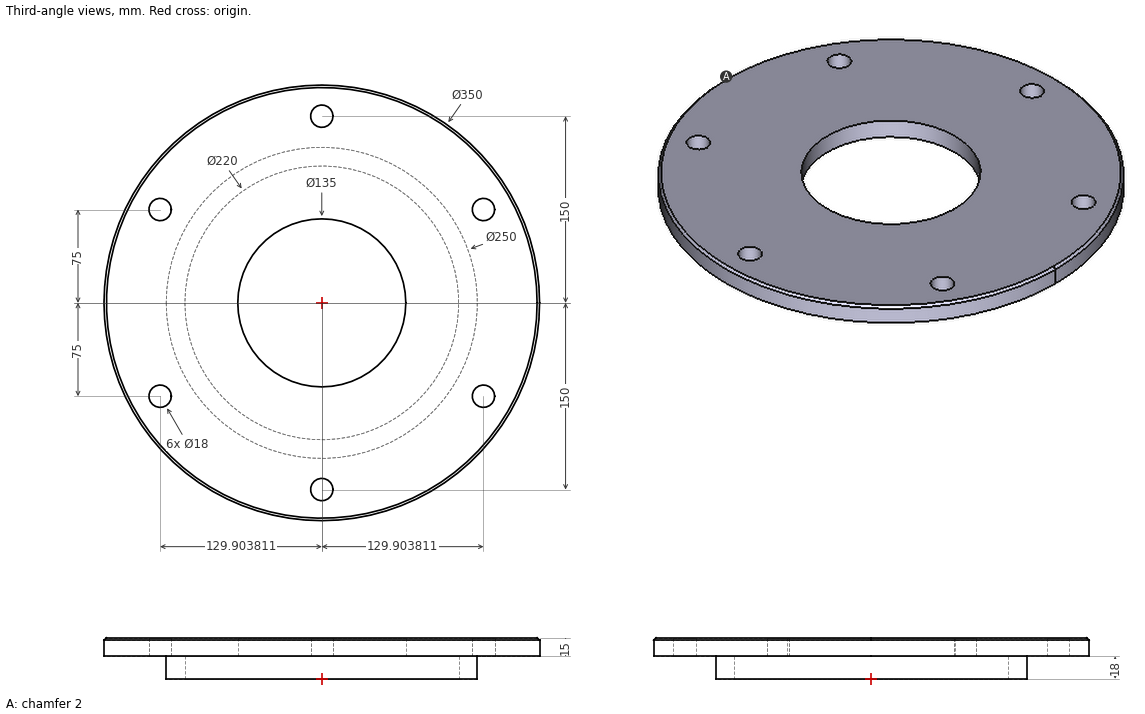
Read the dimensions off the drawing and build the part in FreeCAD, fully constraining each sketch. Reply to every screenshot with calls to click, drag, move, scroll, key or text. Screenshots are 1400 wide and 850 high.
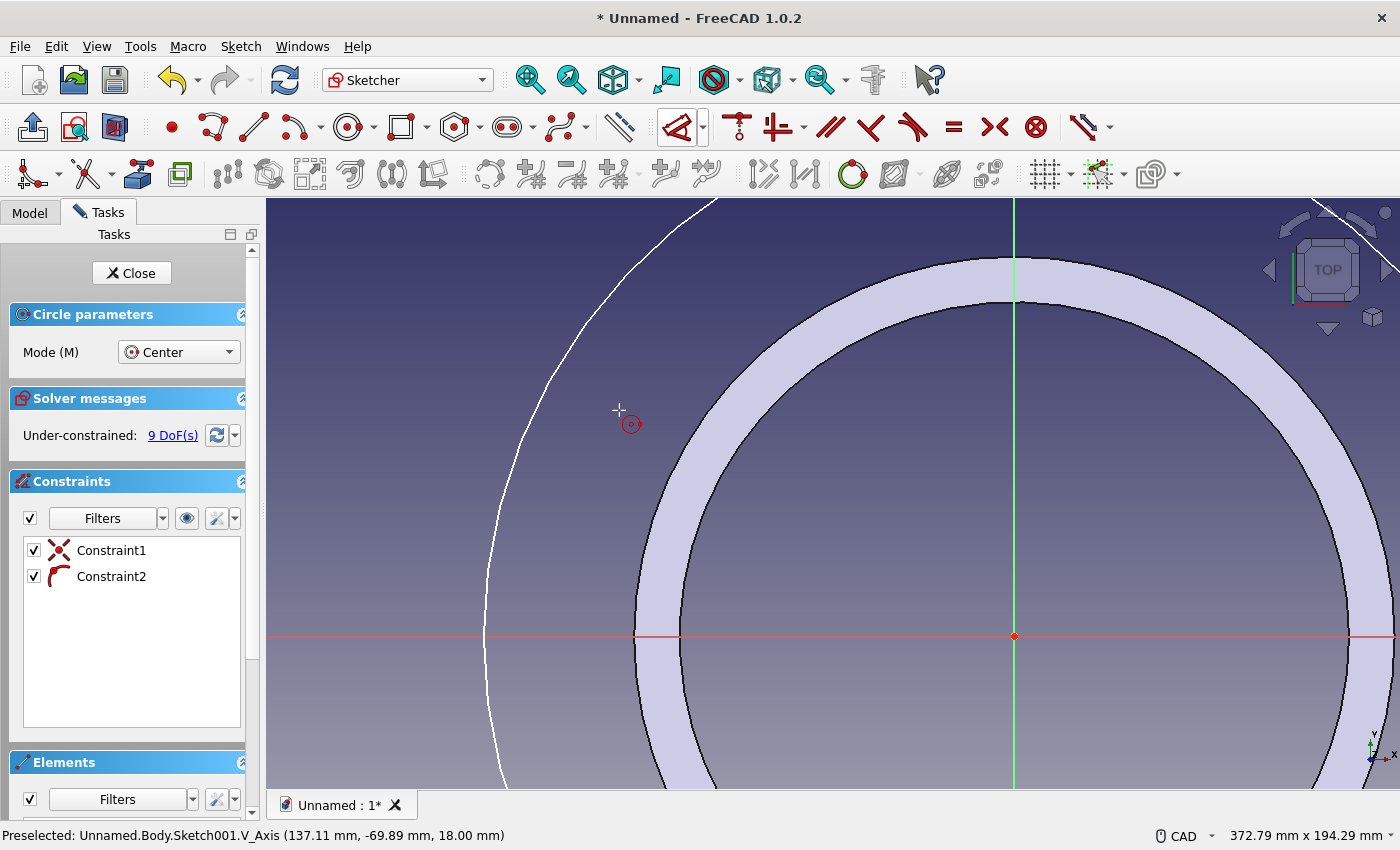
click(619, 409)
click(639, 389)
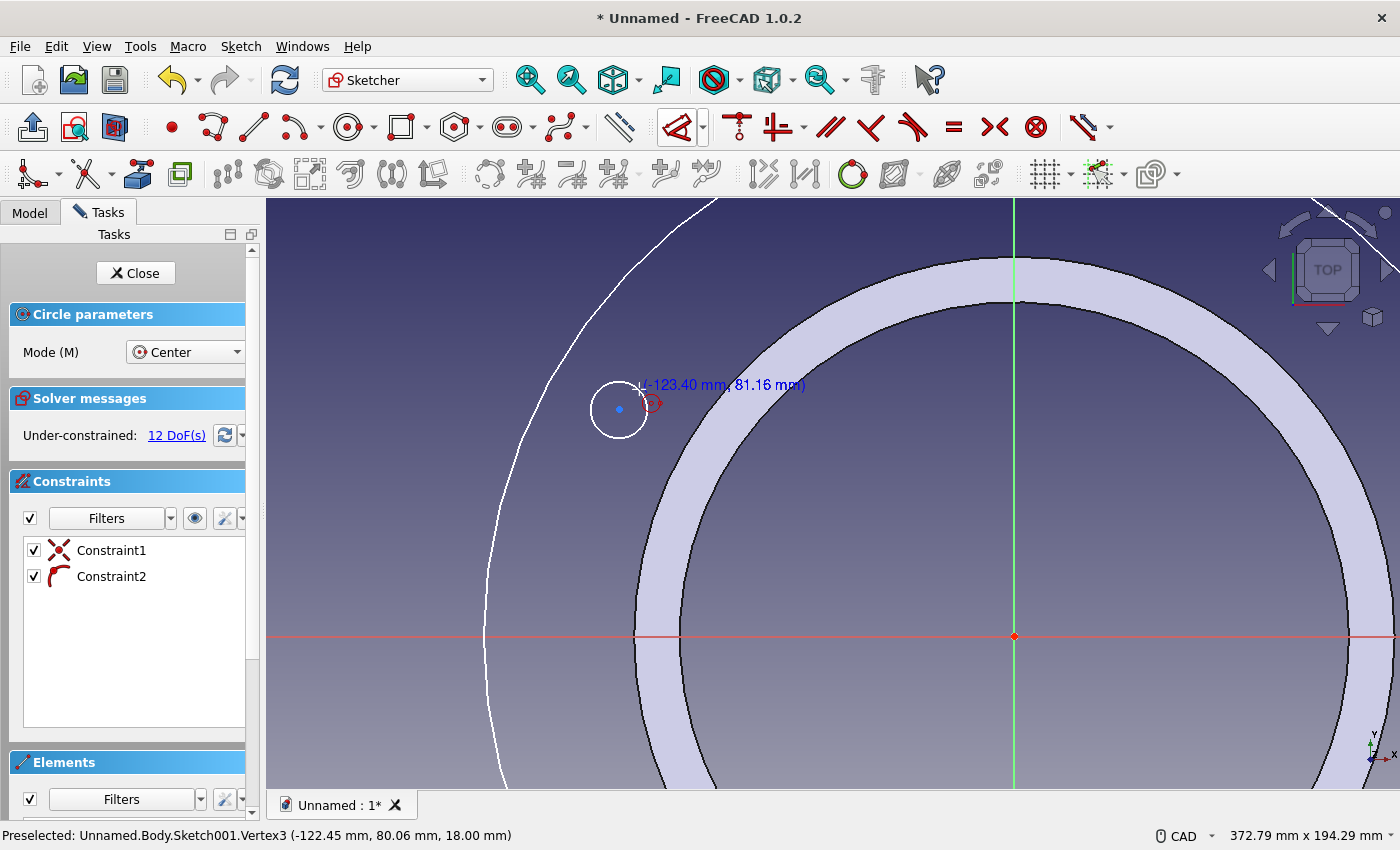
scroll(619, 410, down, 5)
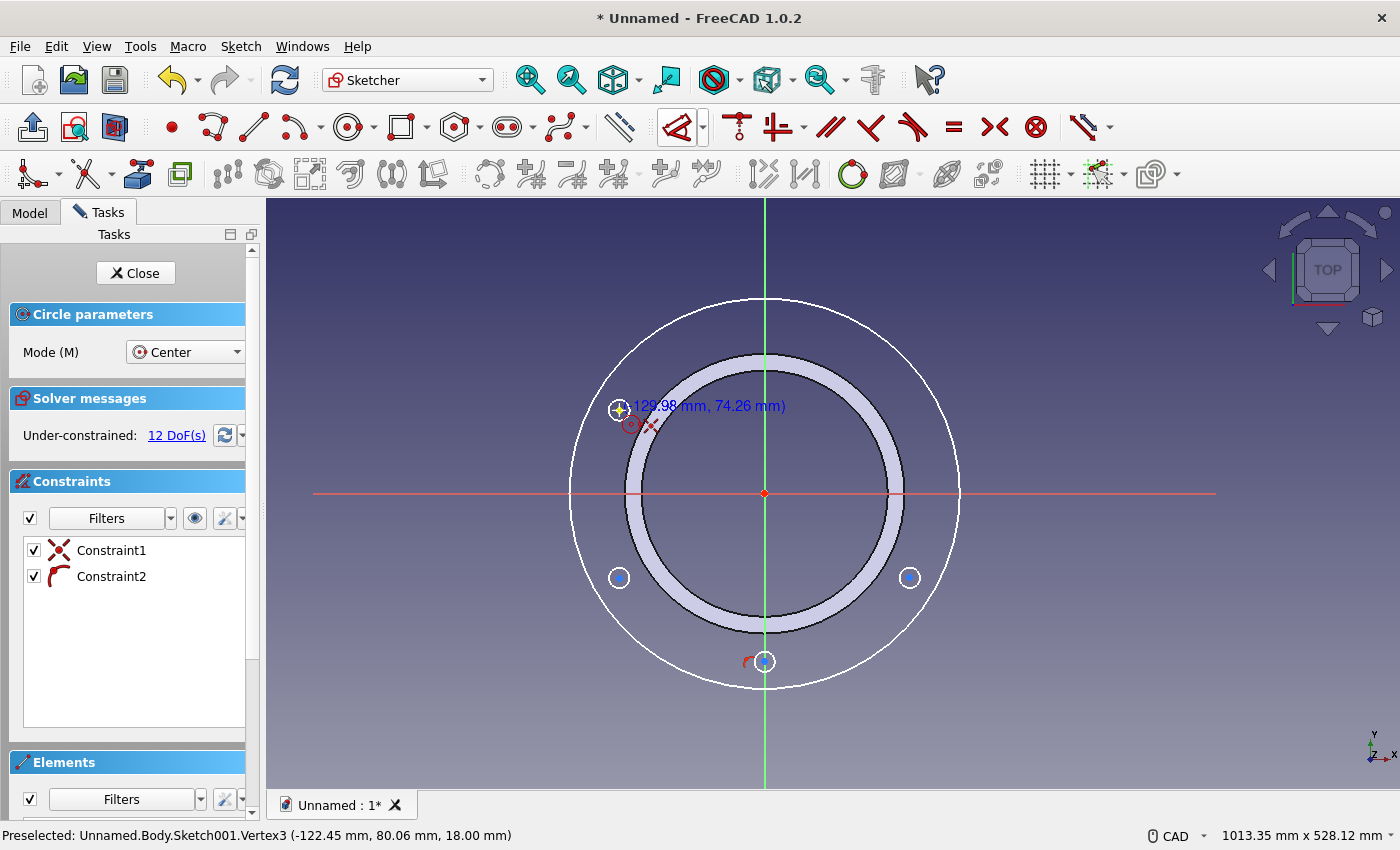
scroll(910, 410, up, 5)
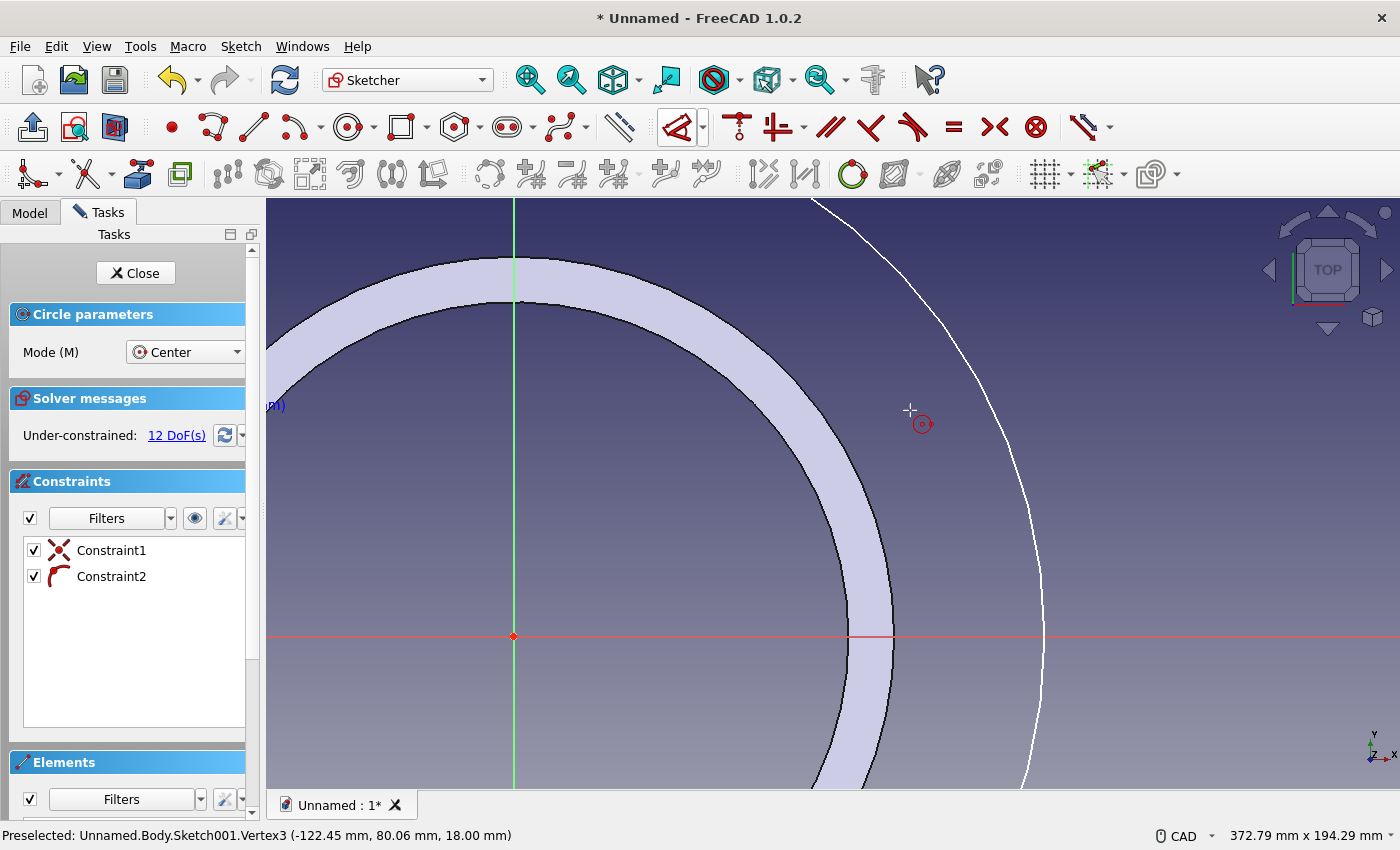
click(909, 409)
click(928, 389)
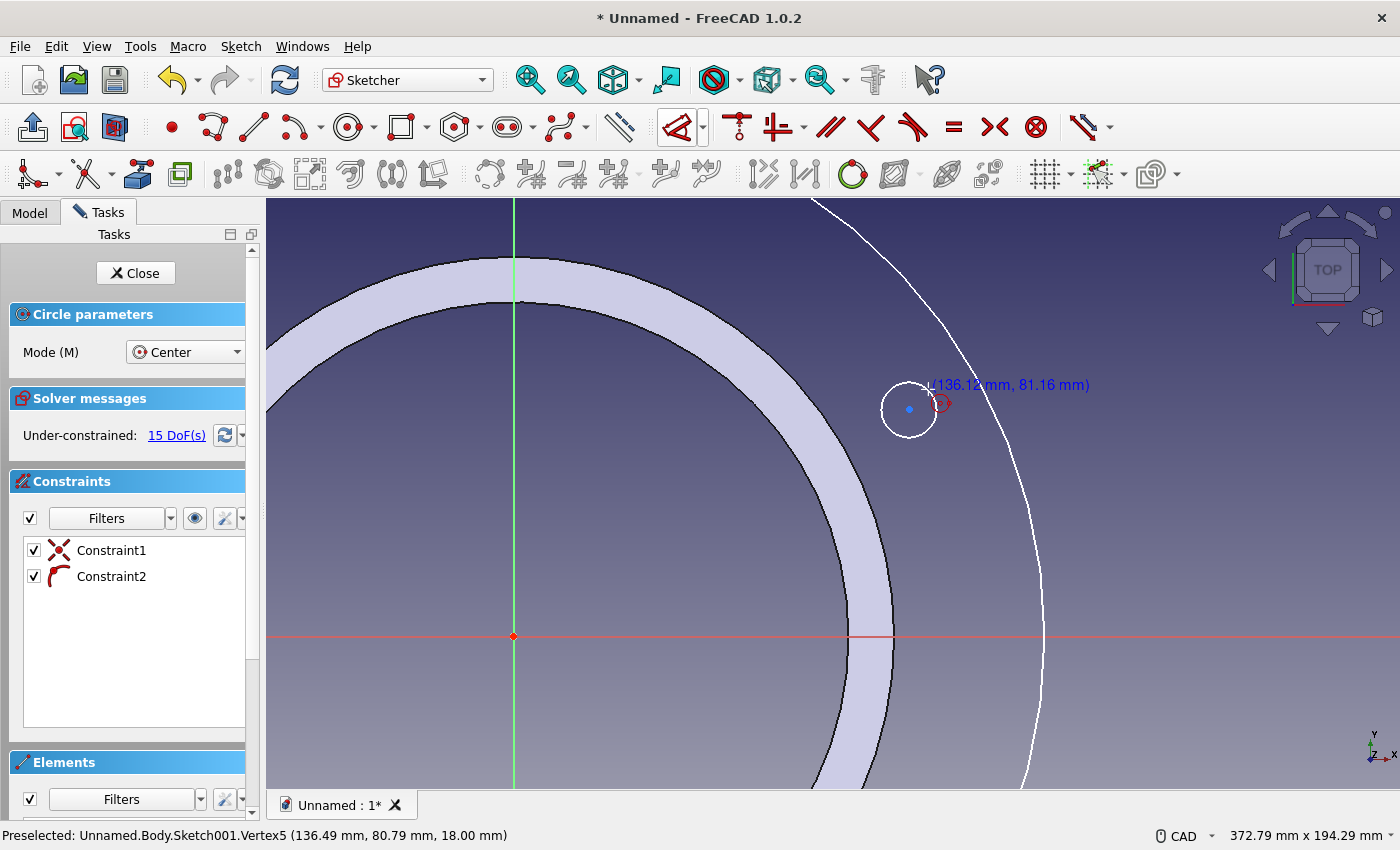
scroll(910, 410, down, 5)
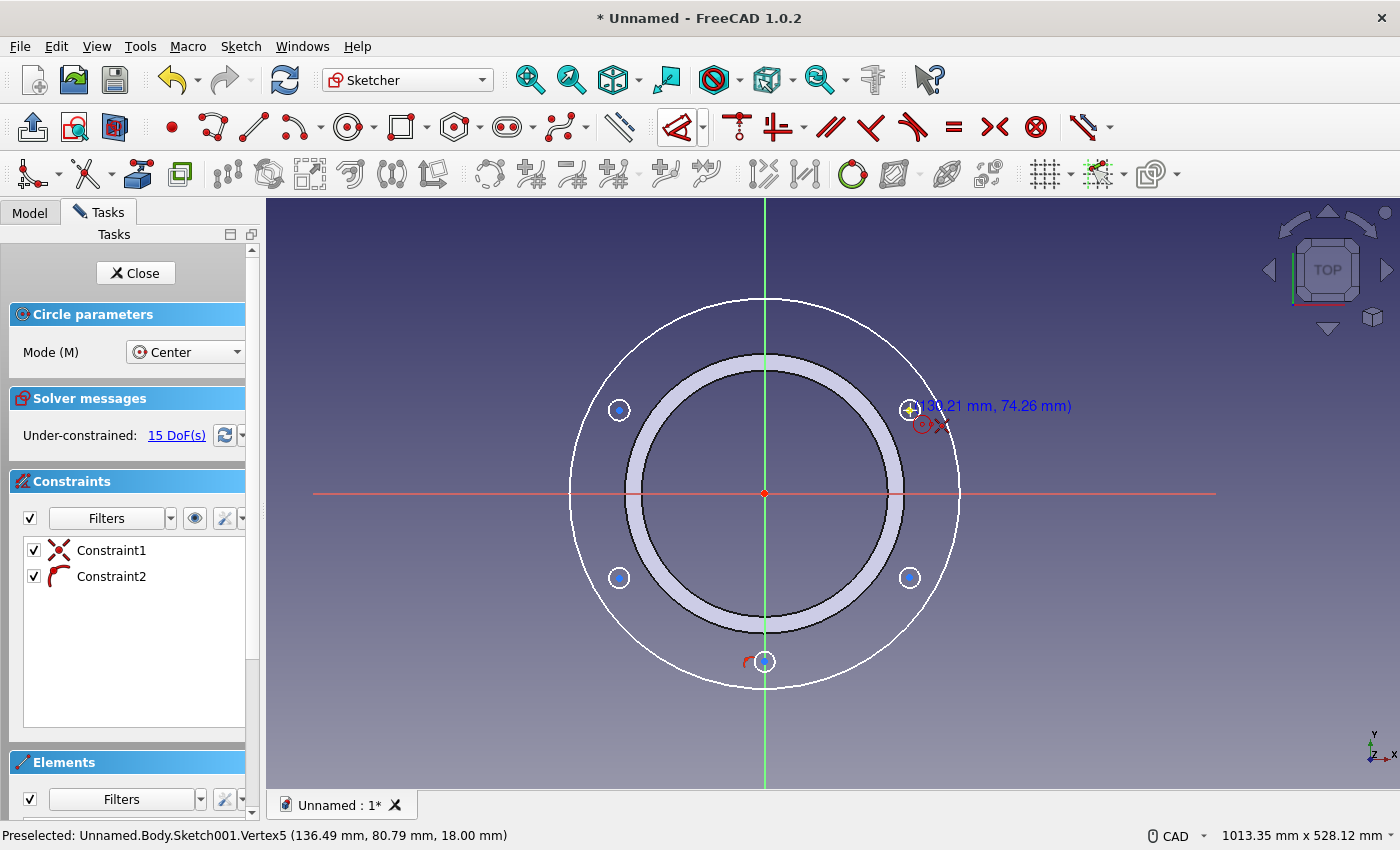
scroll(765, 326, up, 5)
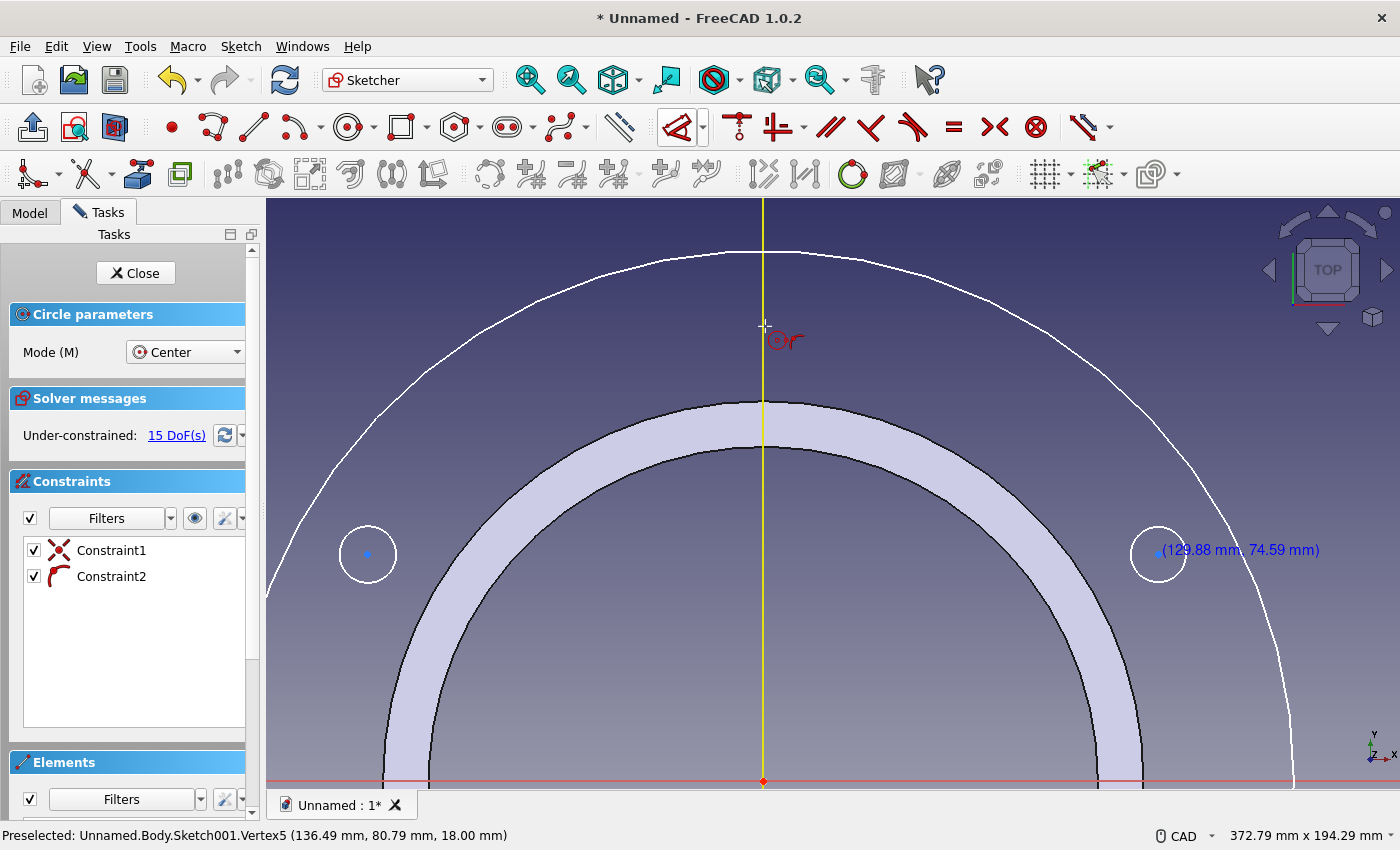
click(763, 325)
click(783, 306)
key(Escape)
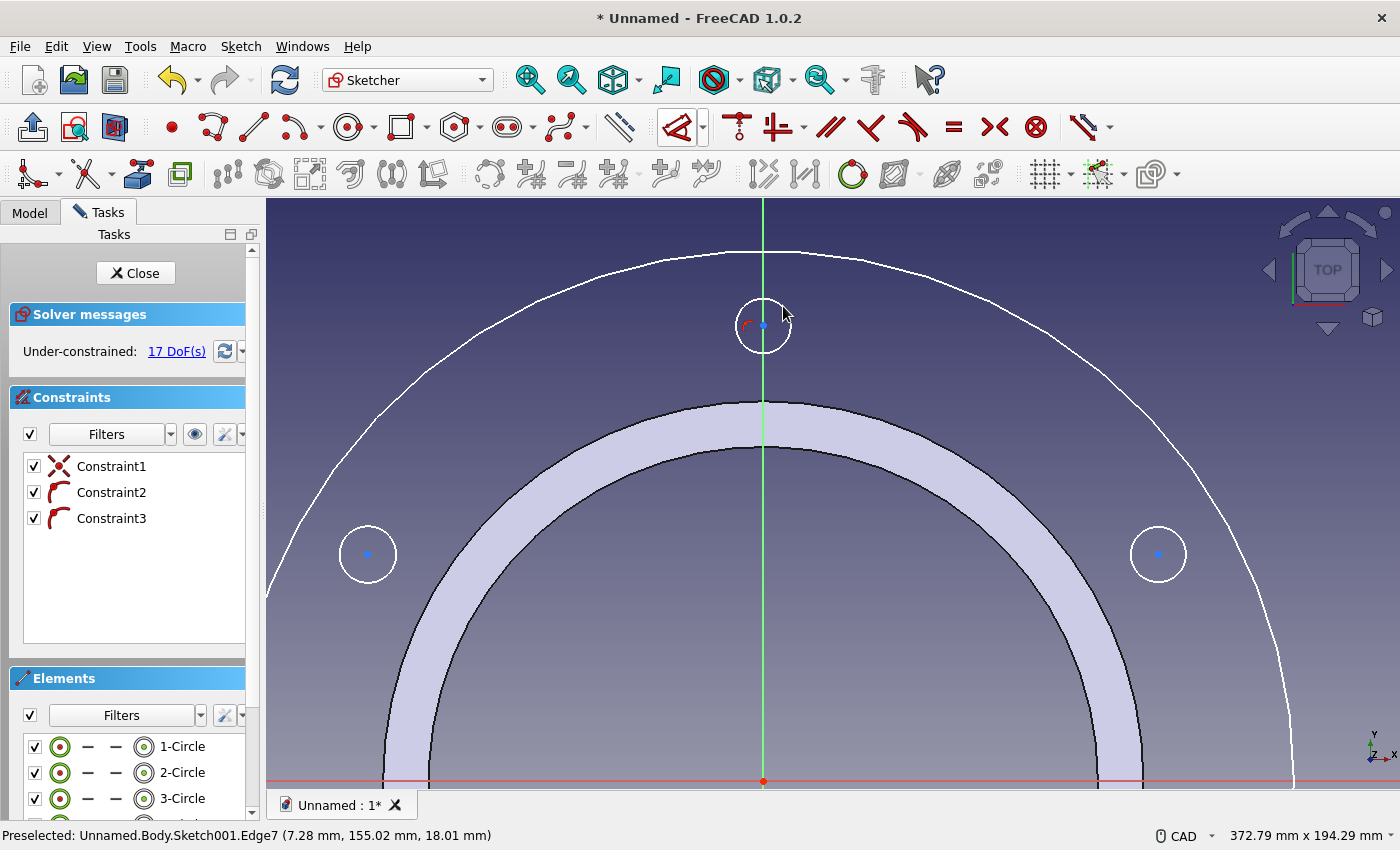
scroll(765, 326, down, 5)